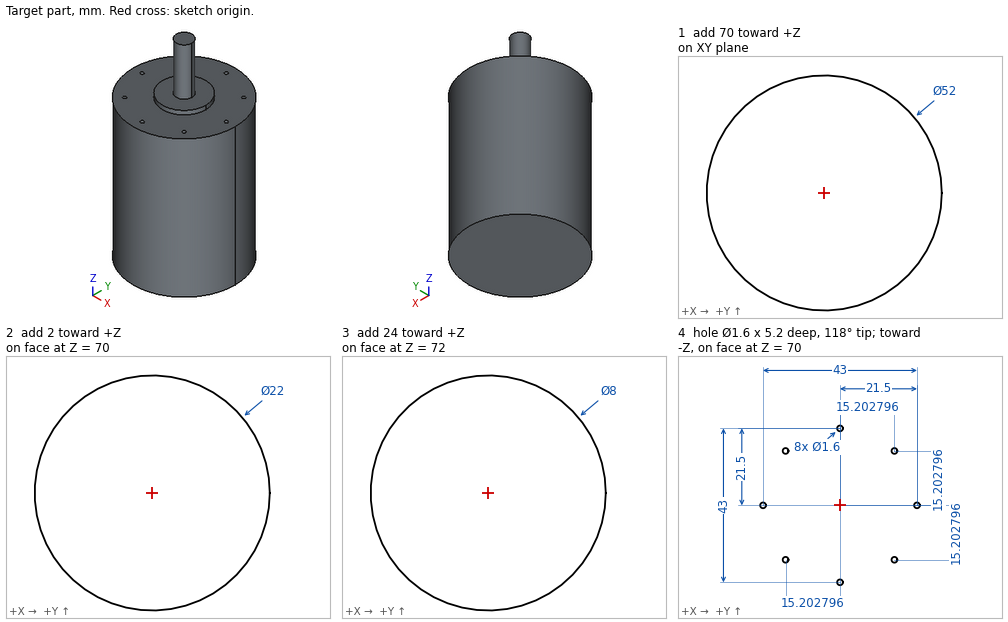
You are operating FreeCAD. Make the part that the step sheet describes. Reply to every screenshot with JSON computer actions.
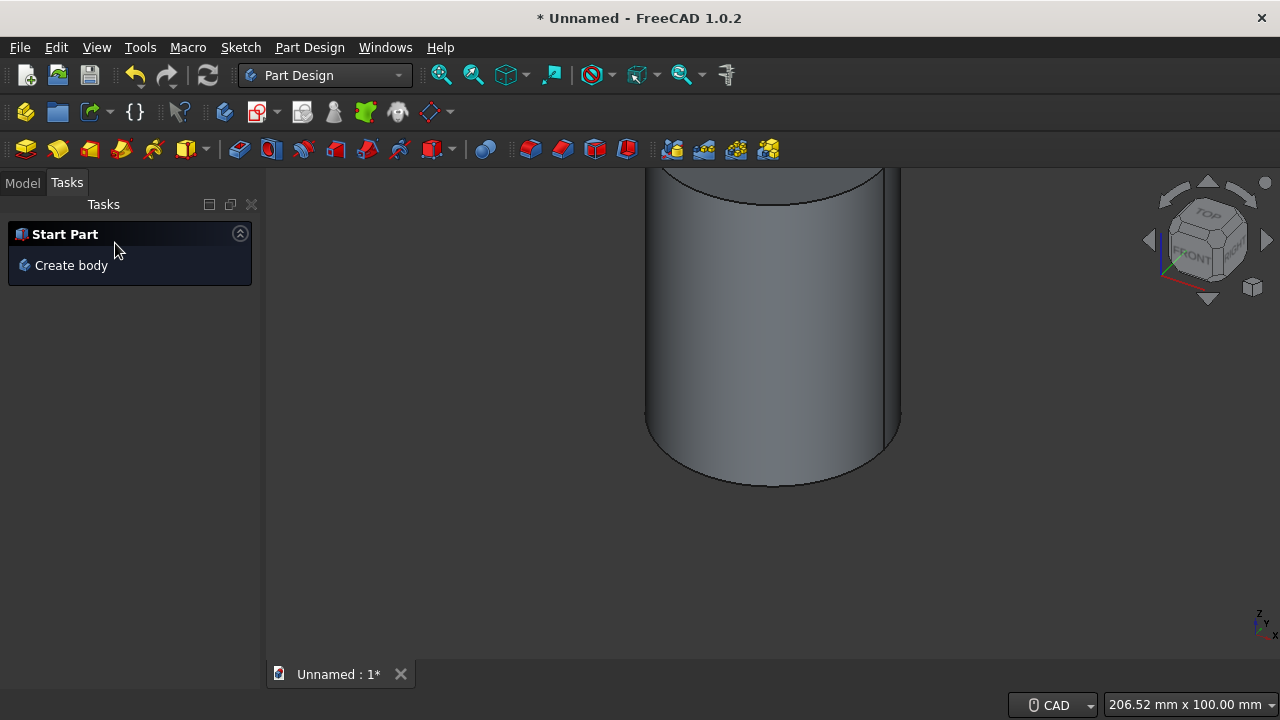
{"action": "left_click", "coordinate": [442, 76]}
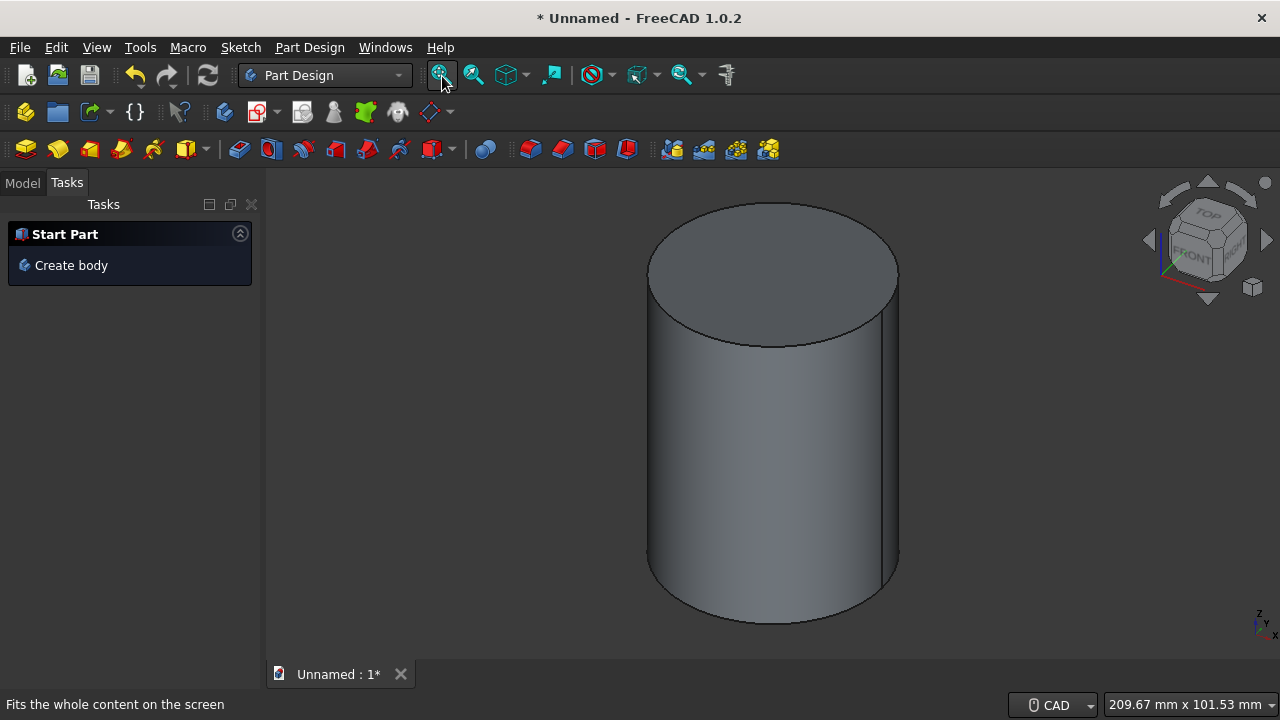
{"action": "left_click", "coordinate": [773, 274]}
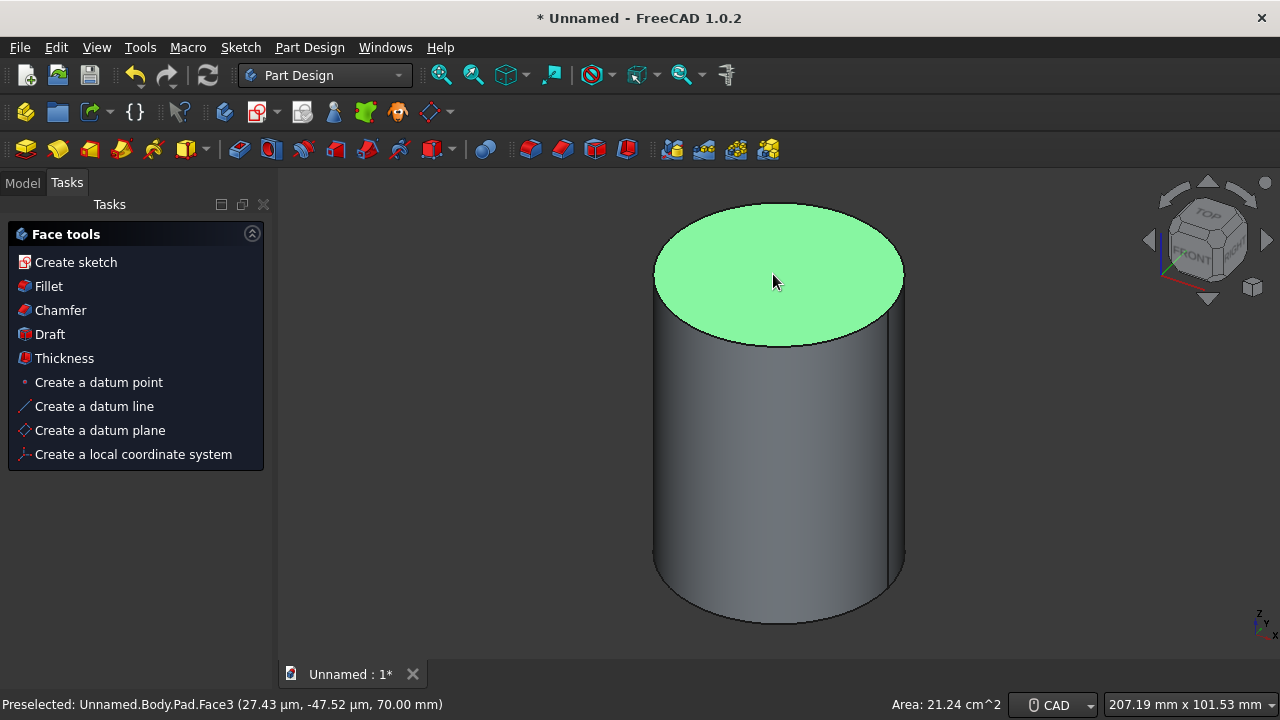
{"action": "left_click", "coordinate": [258, 112]}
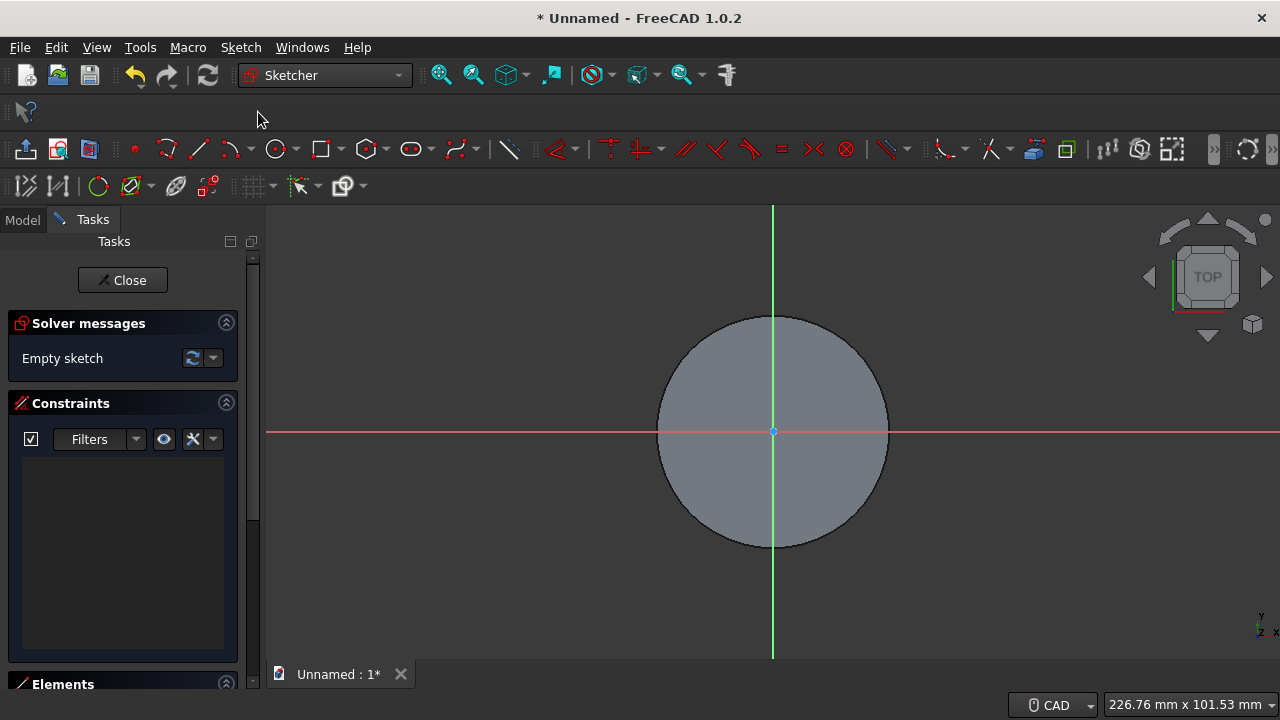
{"action": "scroll", "coordinate": [813, 432], "scroll_direction": "up", "scroll_amount": 5}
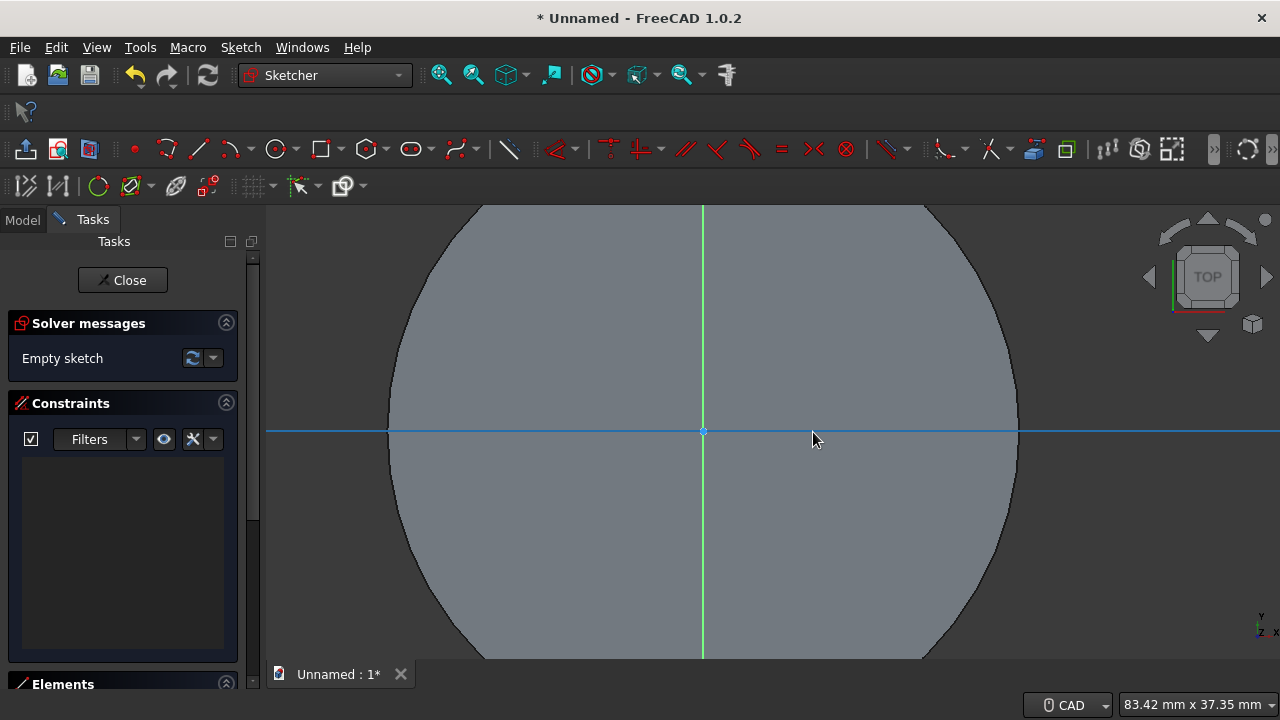
{"action": "left_click", "coordinate": [276, 150]}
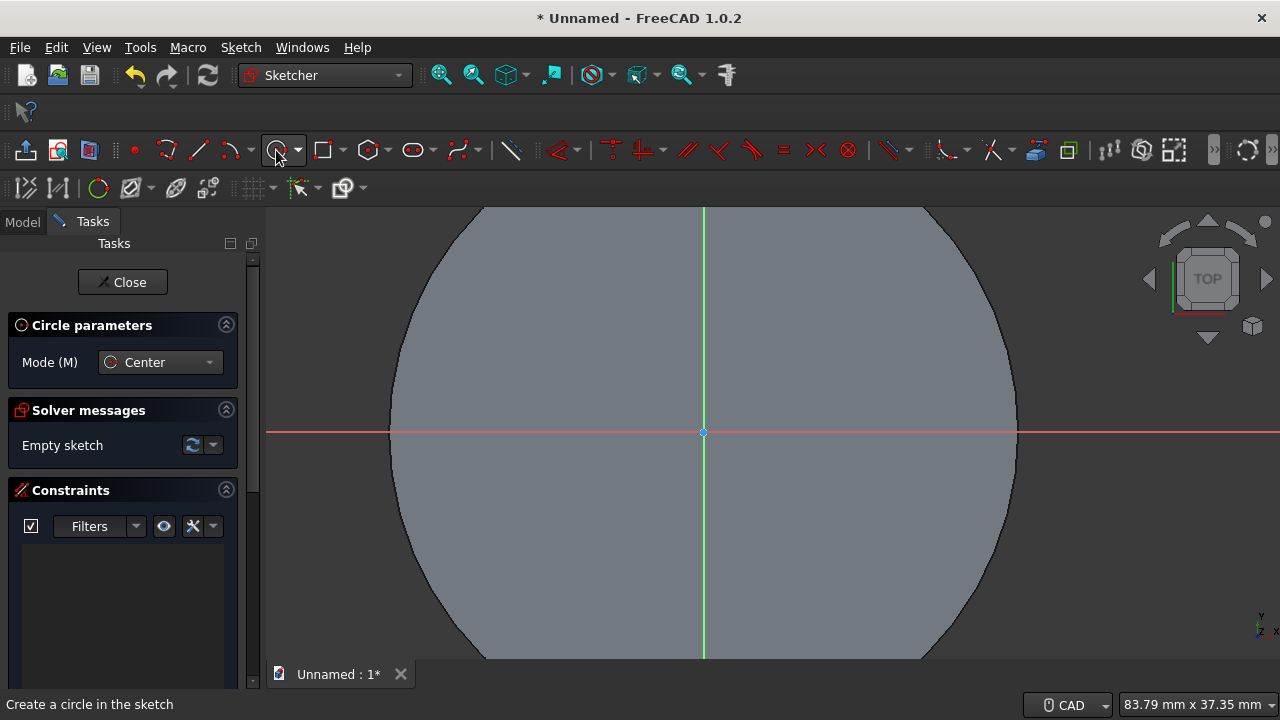
{"action": "left_click", "coordinate": [704, 432]}
{"action": "mouse_move", "coordinate": [798, 338]}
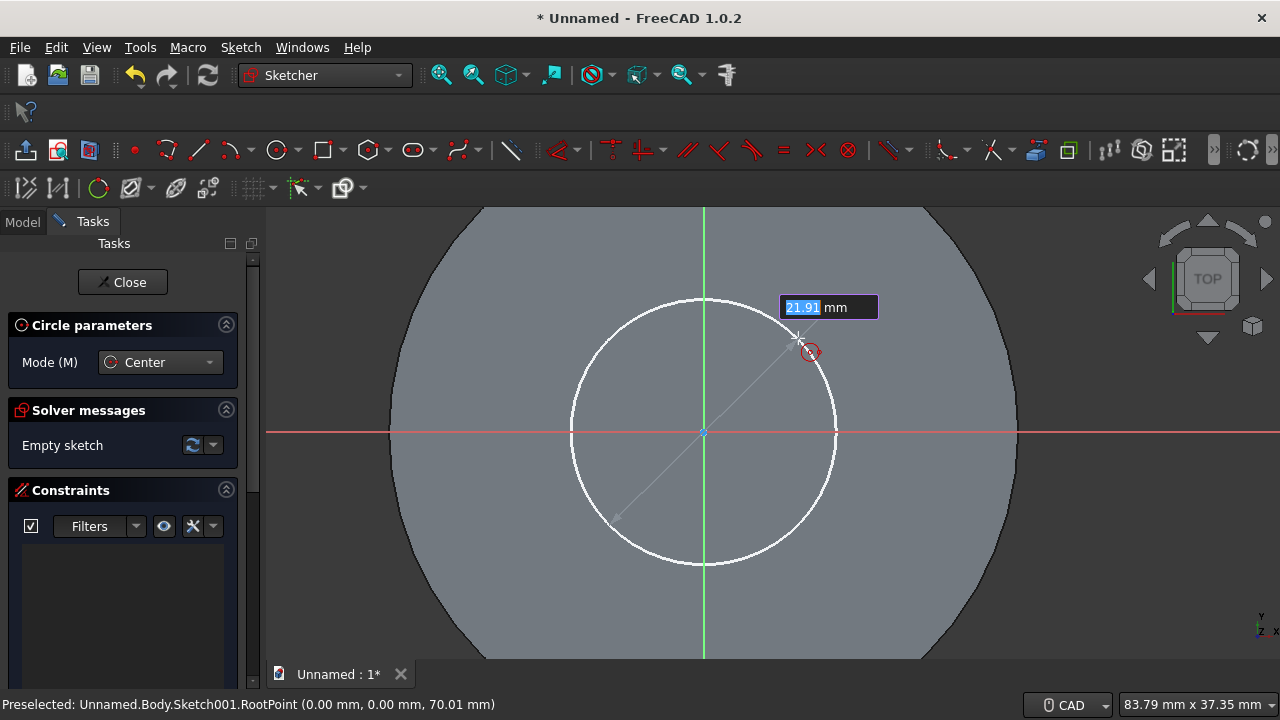
{"action": "type", "text": "22"}
{"action": "key", "text": "Return"}
{"action": "key", "text": "Escape"}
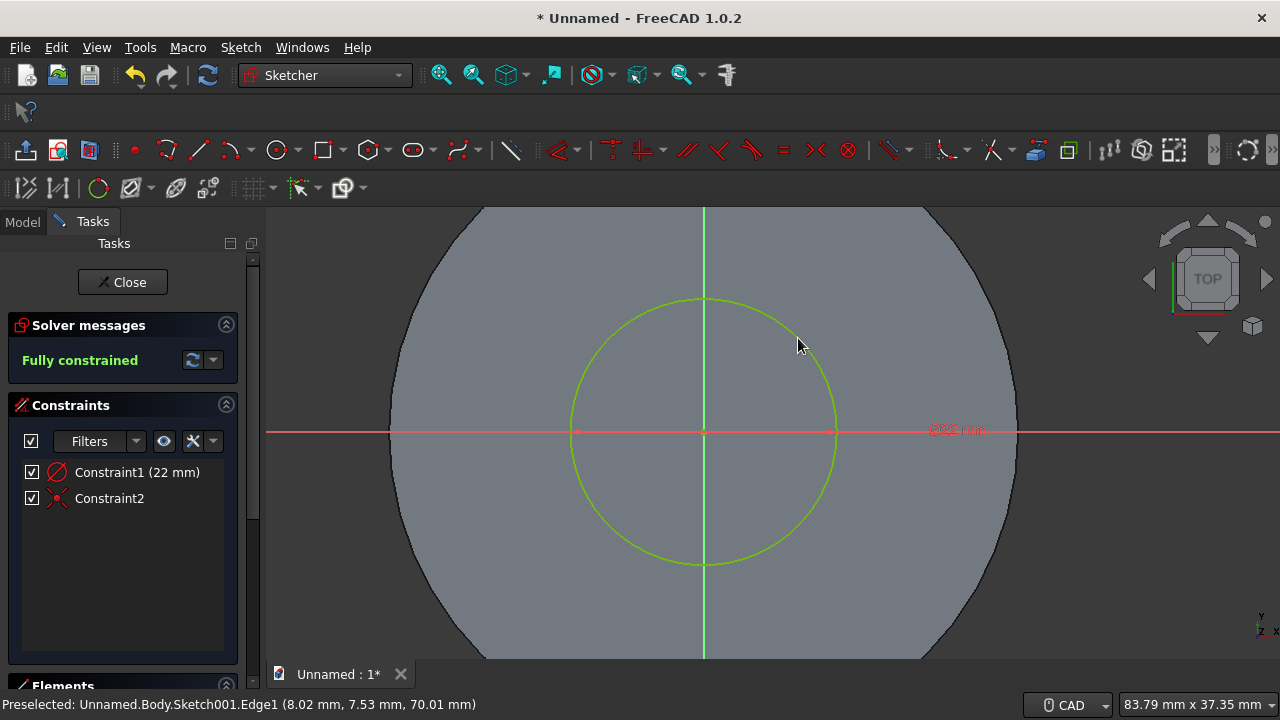
{"action": "left_click", "coordinate": [123, 282]}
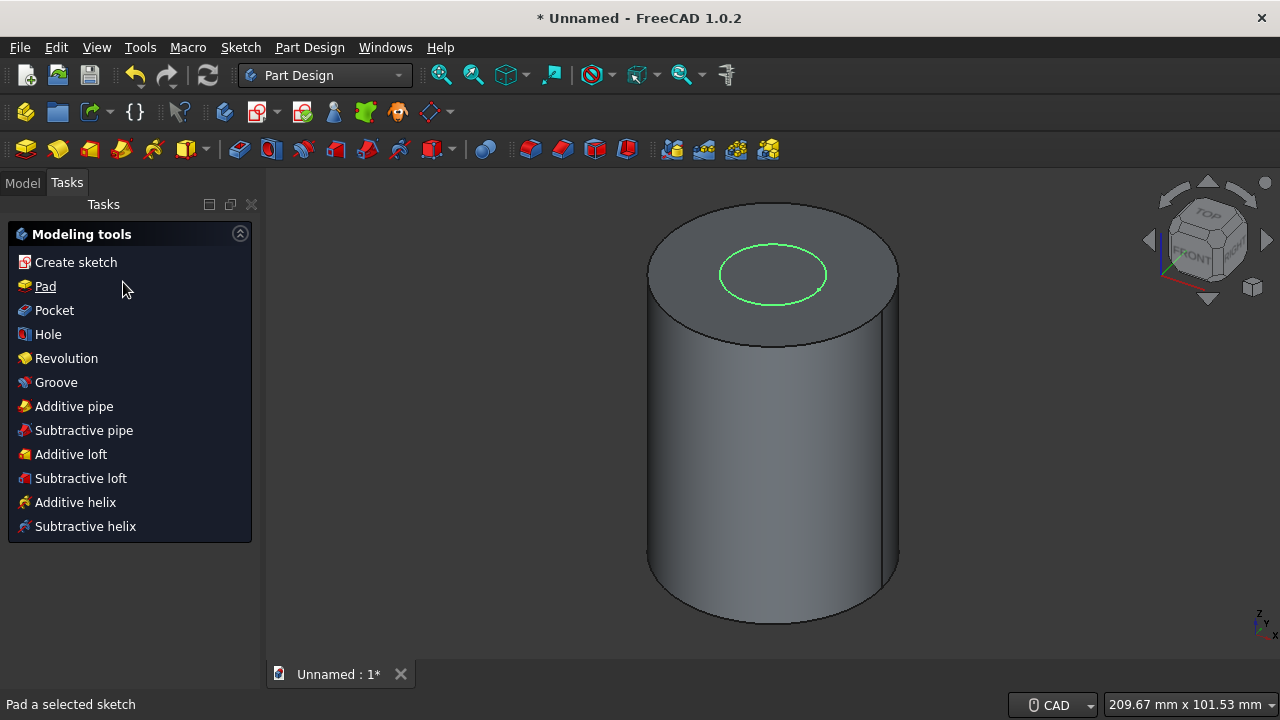
{"action": "left_click", "coordinate": [26, 150]}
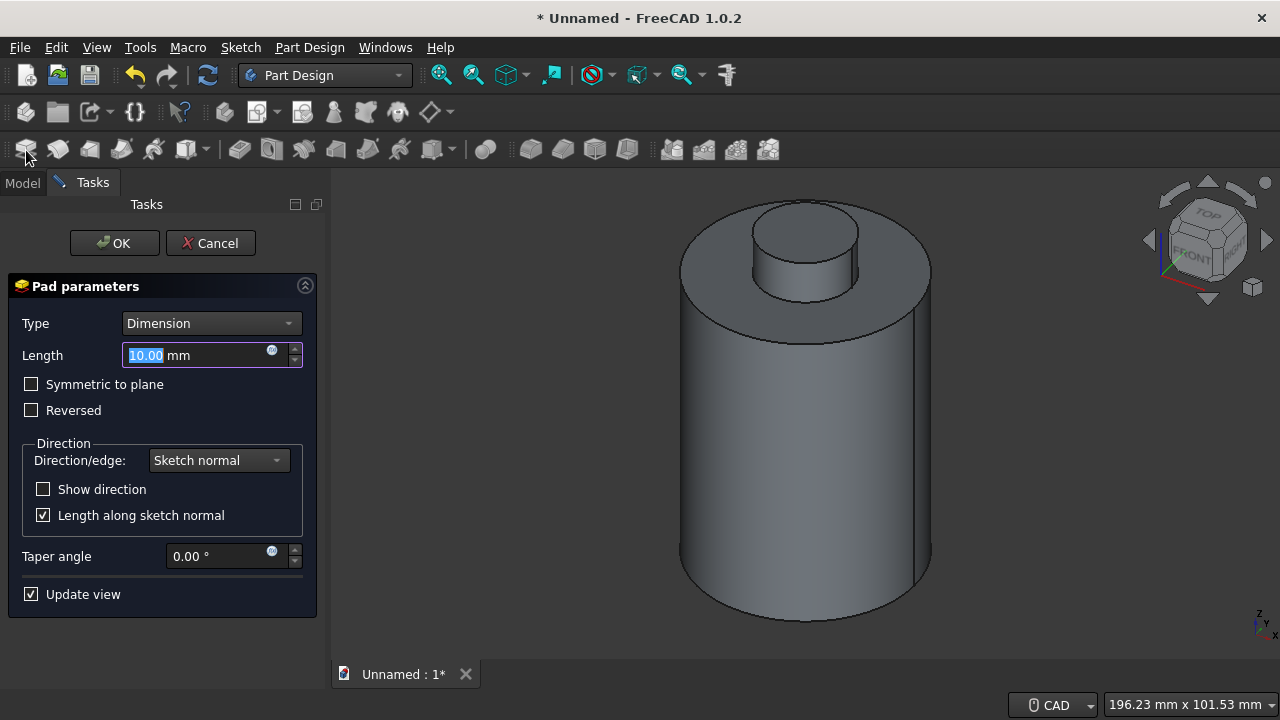
{"action": "type", "text": "2"}
{"action": "key", "text": "Tab"}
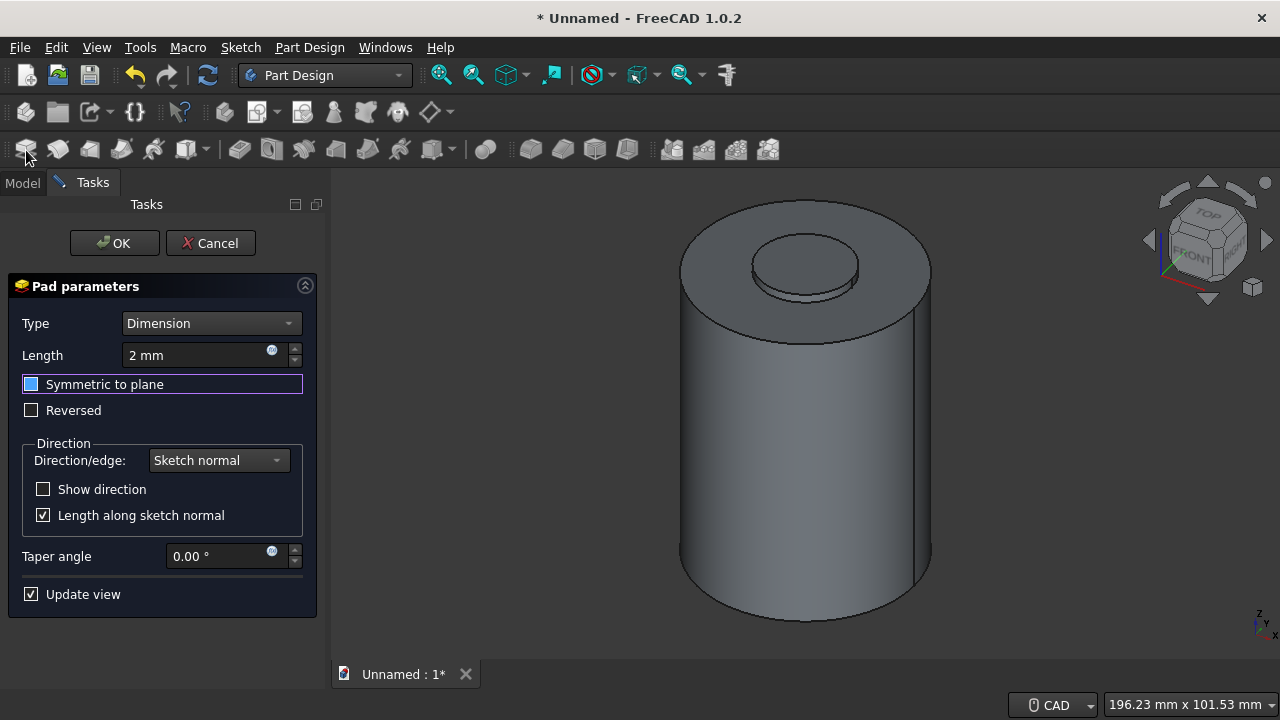
{"action": "left_click", "coordinate": [115, 243]}